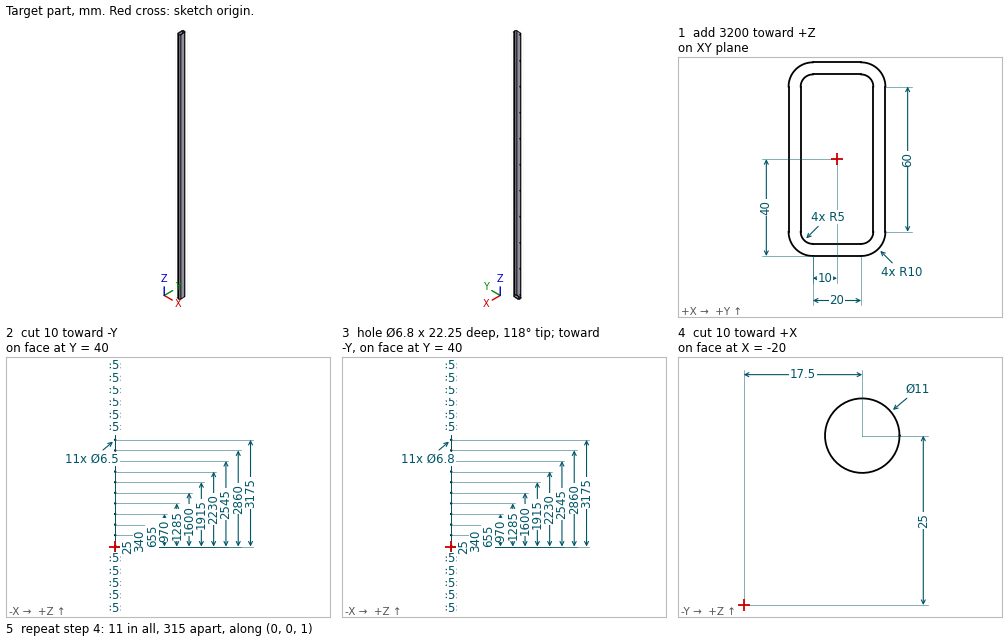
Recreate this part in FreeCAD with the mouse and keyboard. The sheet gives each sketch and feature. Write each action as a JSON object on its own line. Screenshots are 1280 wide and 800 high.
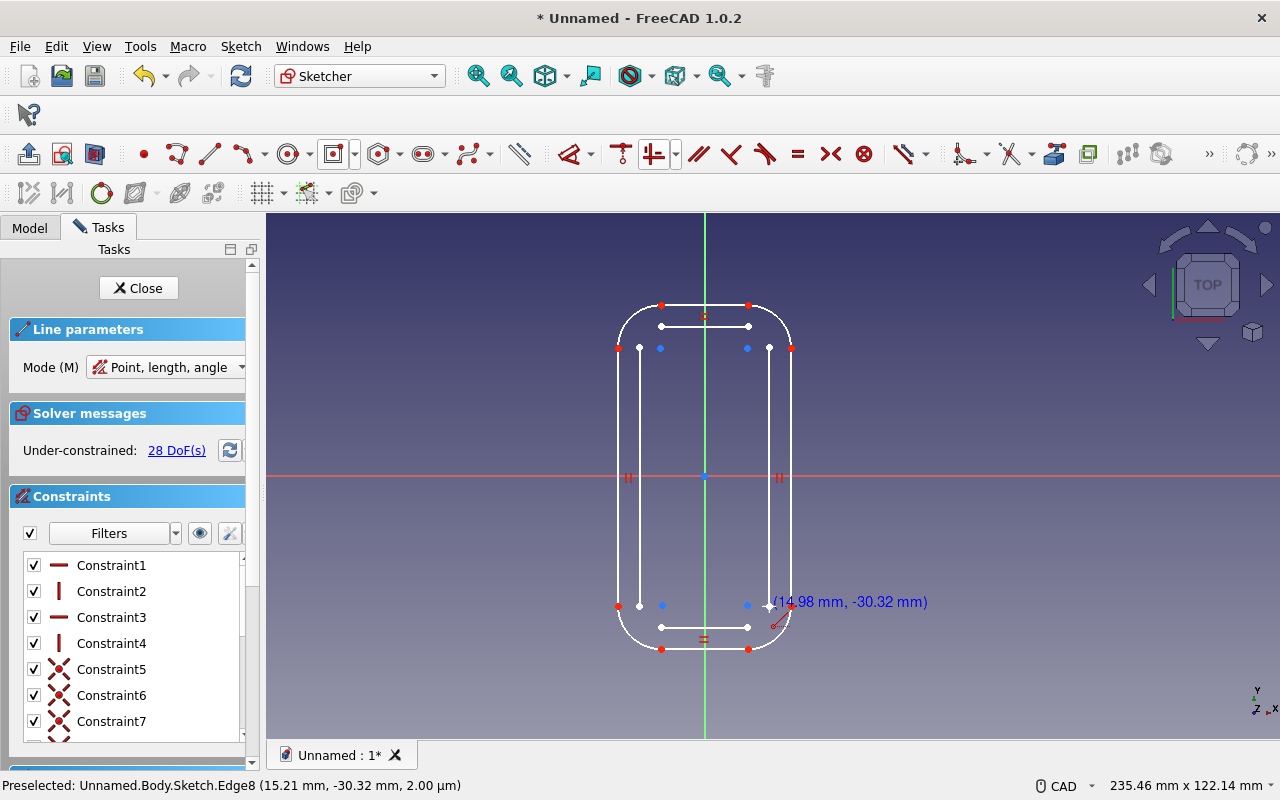
{"action": "left_click", "coordinate": [242, 154]}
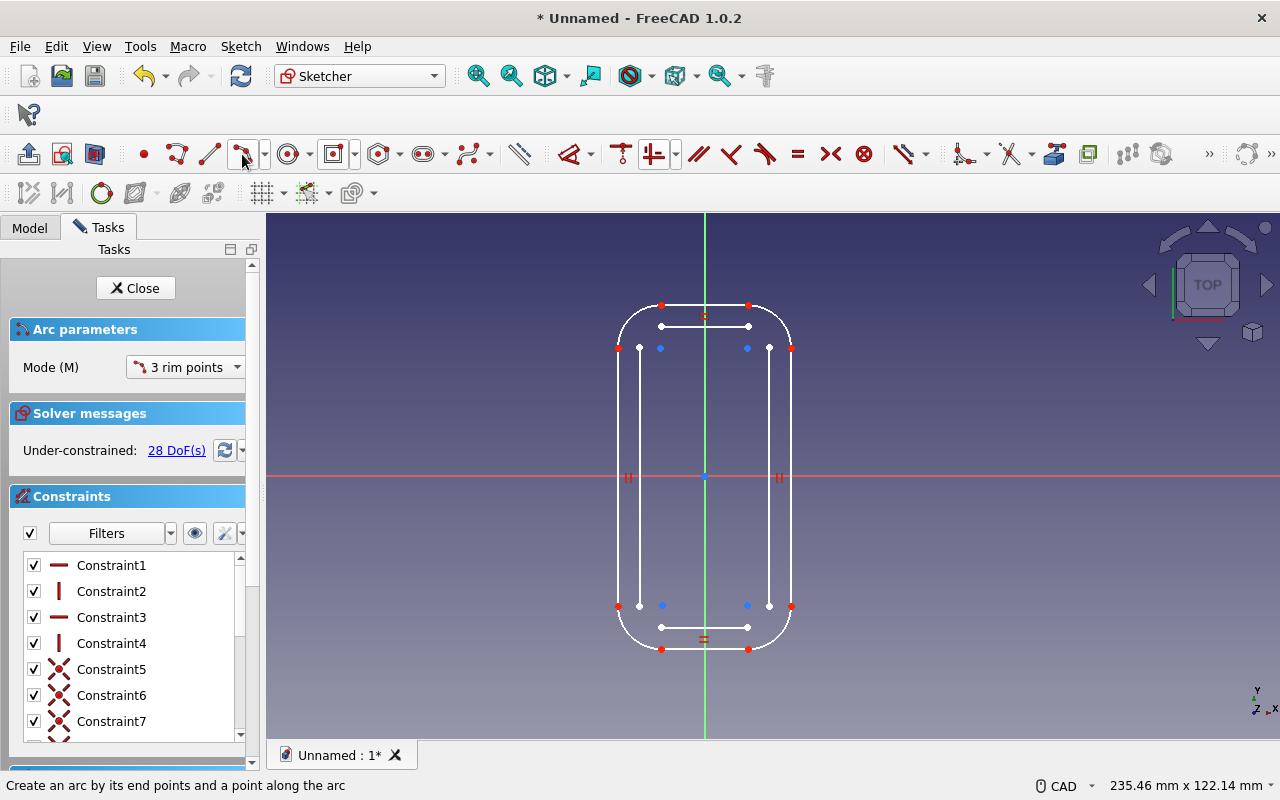
{"action": "left_click", "coordinate": [661, 628]}
{"action": "left_click", "coordinate": [640, 606]}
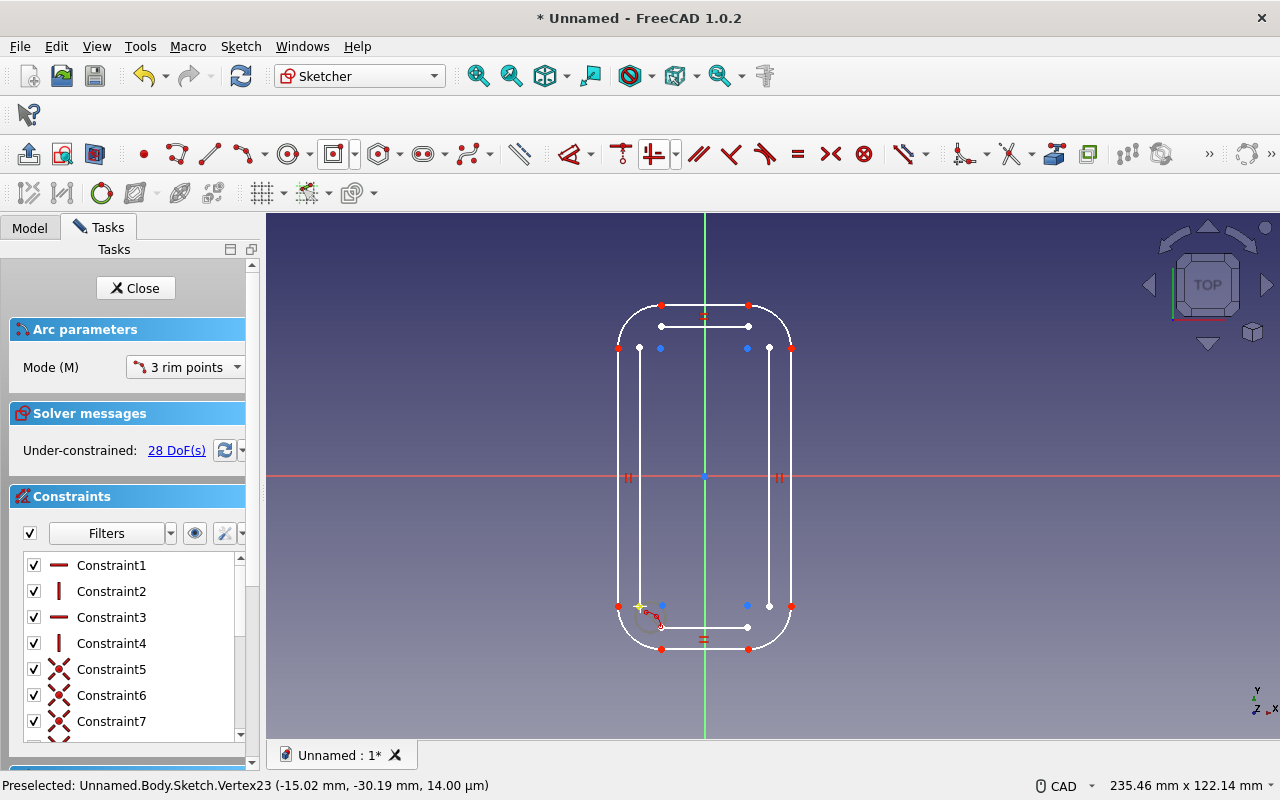
{"action": "scroll", "coordinate": [646, 621], "scroll_direction": "up", "scroll_amount": 5}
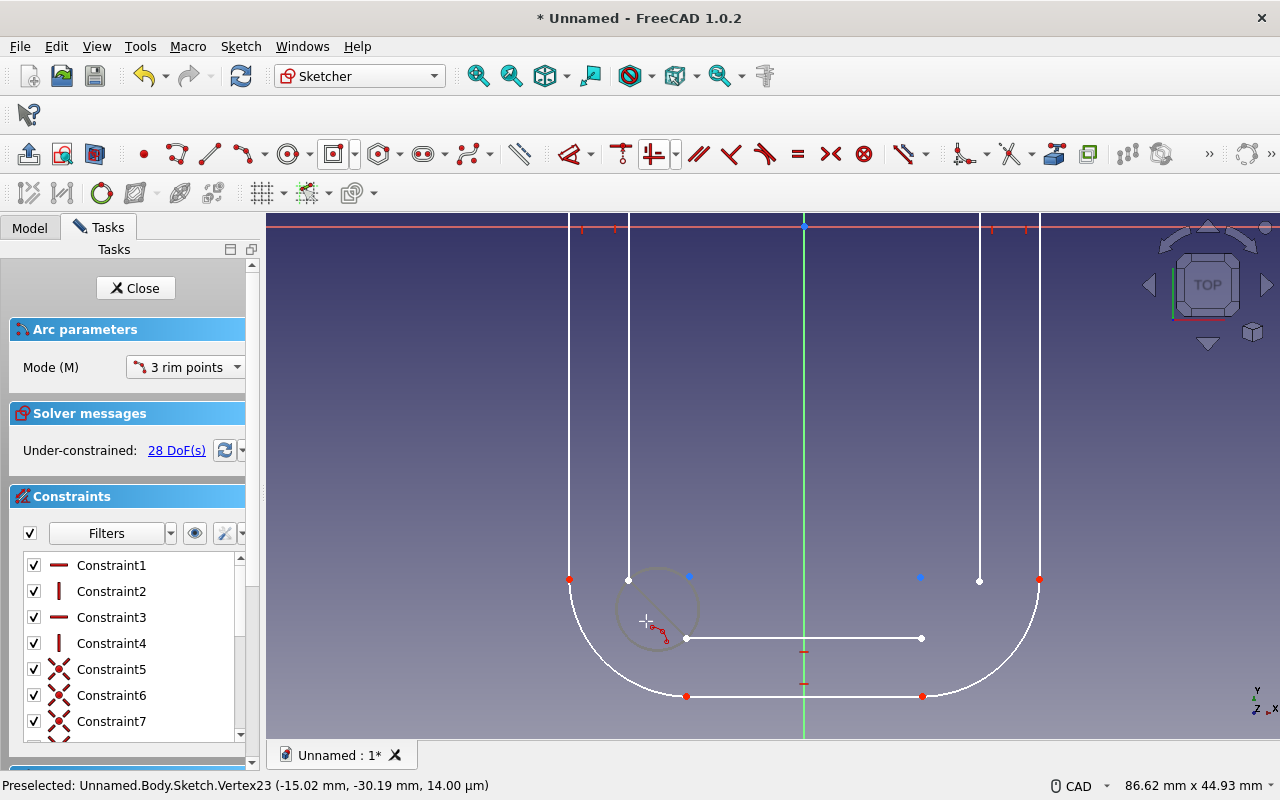
{"action": "left_click", "coordinate": [646, 619]}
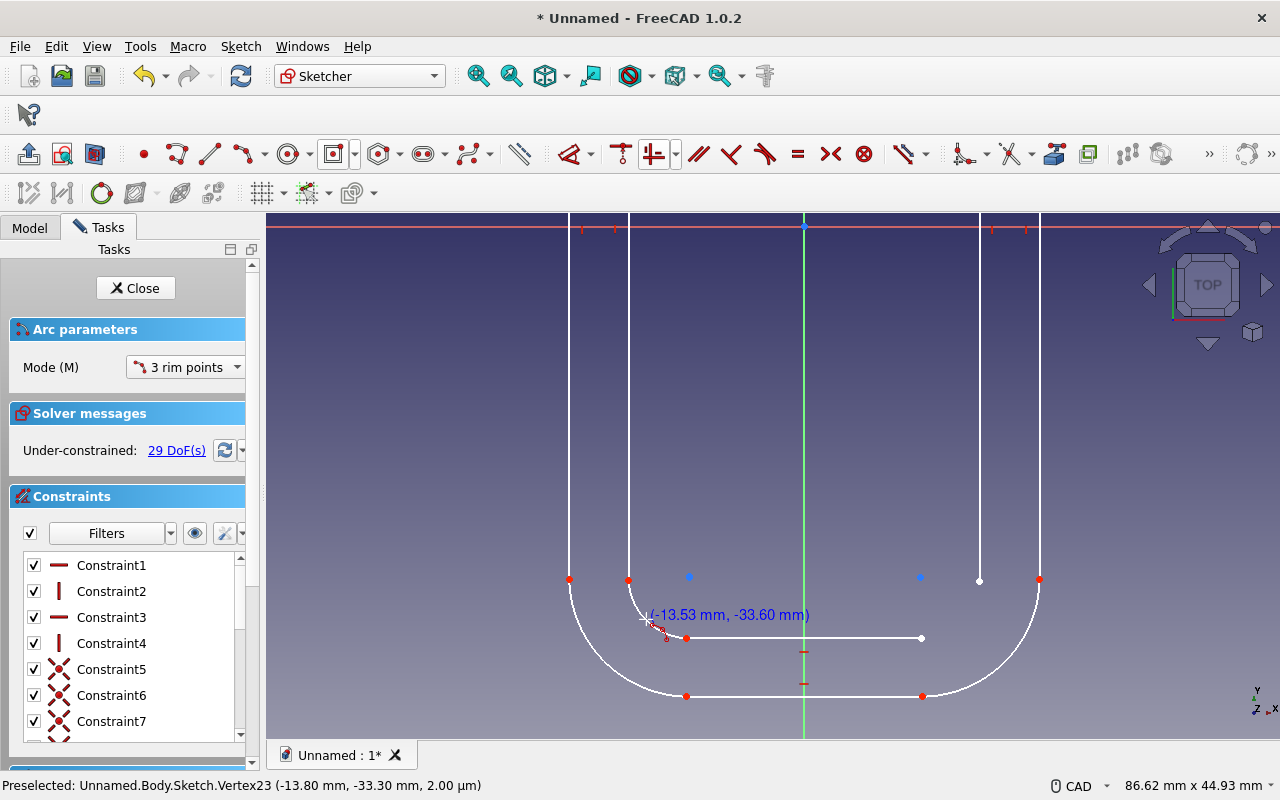
{"action": "scroll", "coordinate": [646, 621], "scroll_direction": "down", "scroll_amount": 5}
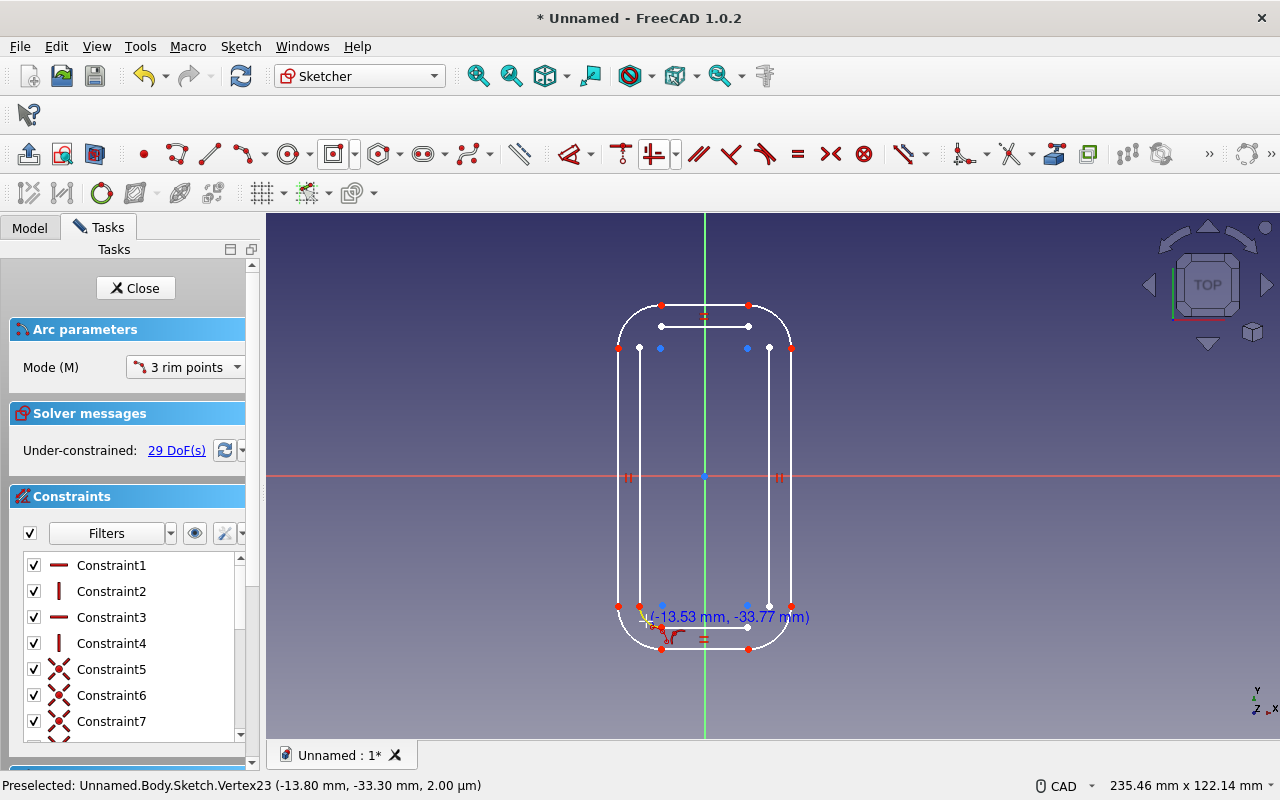
{"action": "left_click", "coordinate": [640, 348]}
{"action": "left_click", "coordinate": [661, 327]}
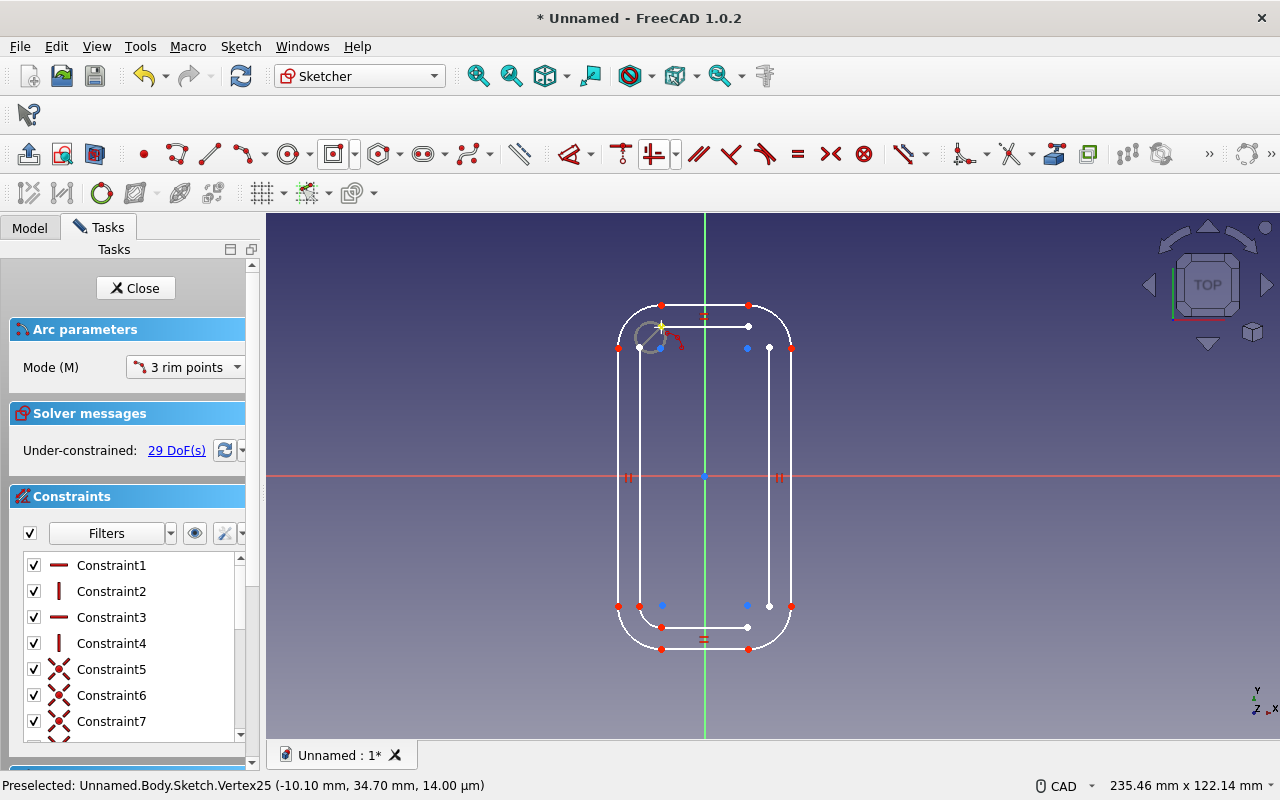
{"action": "scroll", "coordinate": [646, 332], "scroll_direction": "up", "scroll_amount": 5}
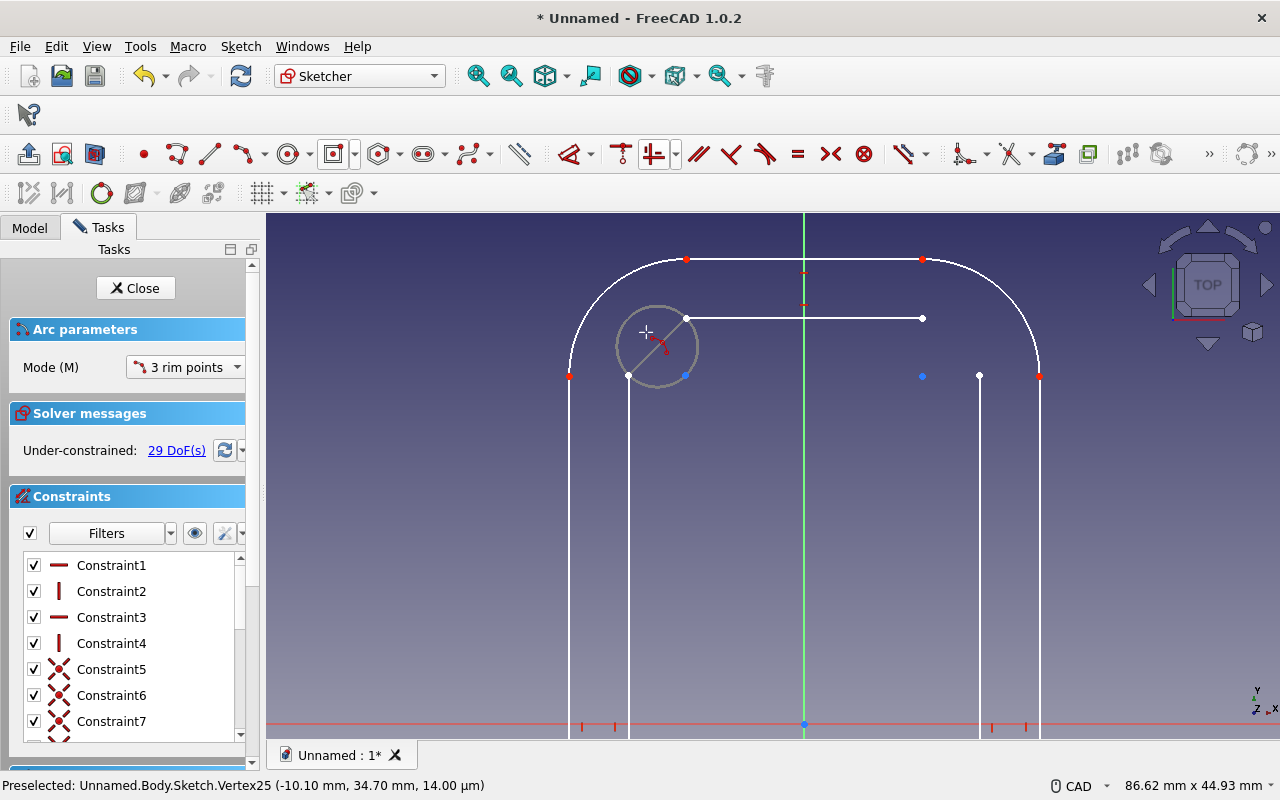
{"action": "left_click", "coordinate": [646, 332]}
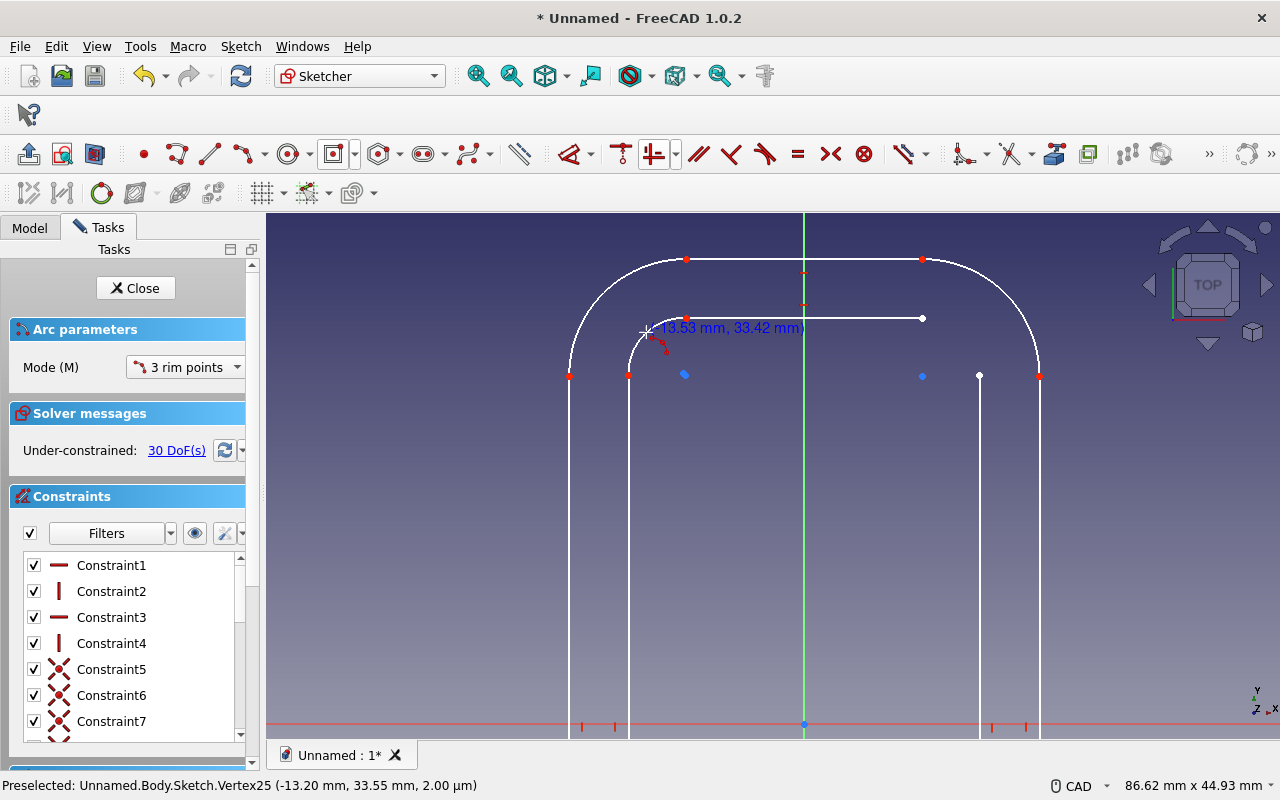
{"action": "left_click", "coordinate": [923, 318]}
{"action": "left_click", "coordinate": [980, 375]}
{"action": "left_click", "coordinate": [963, 332]}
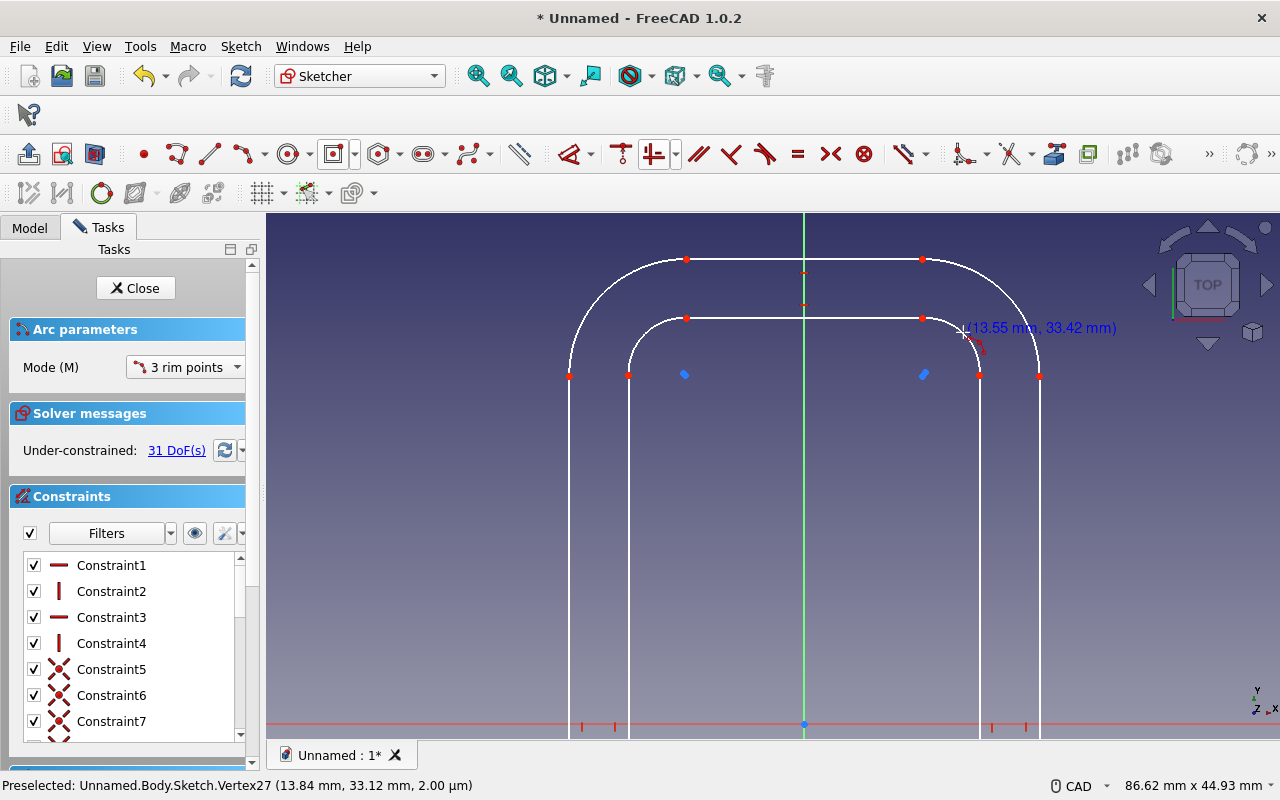
{"action": "scroll", "coordinate": [646, 332], "scroll_direction": "down", "scroll_amount": 5}